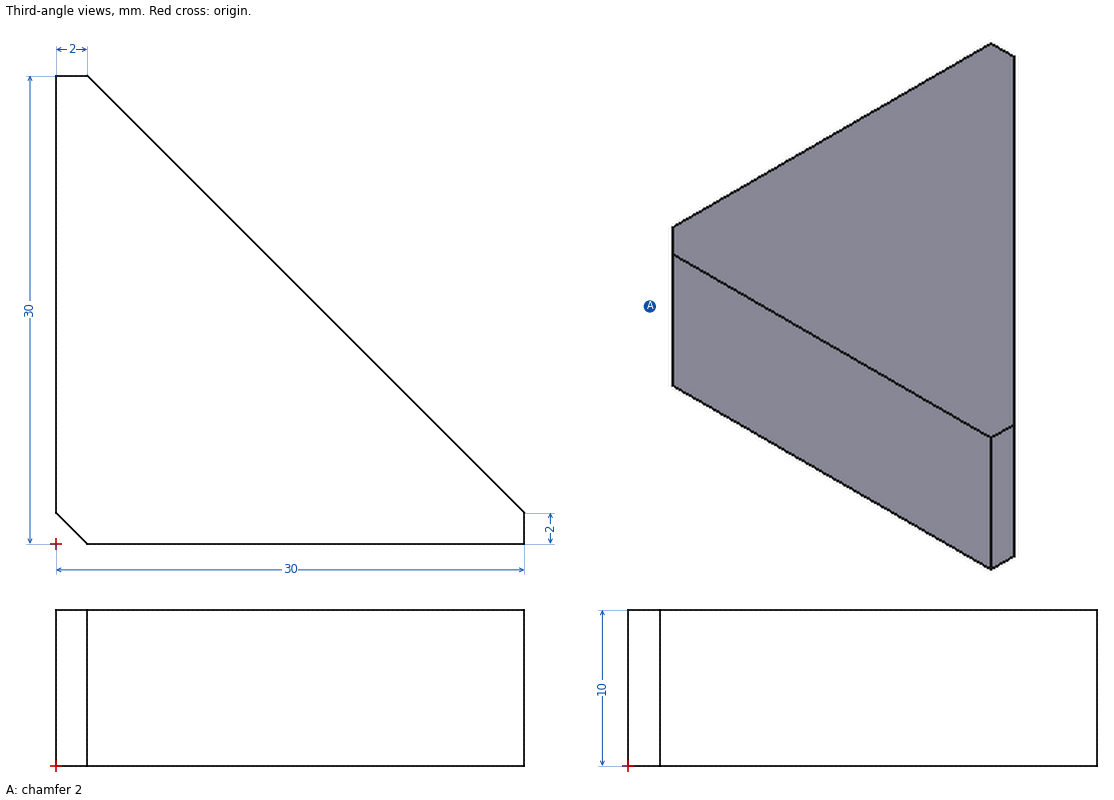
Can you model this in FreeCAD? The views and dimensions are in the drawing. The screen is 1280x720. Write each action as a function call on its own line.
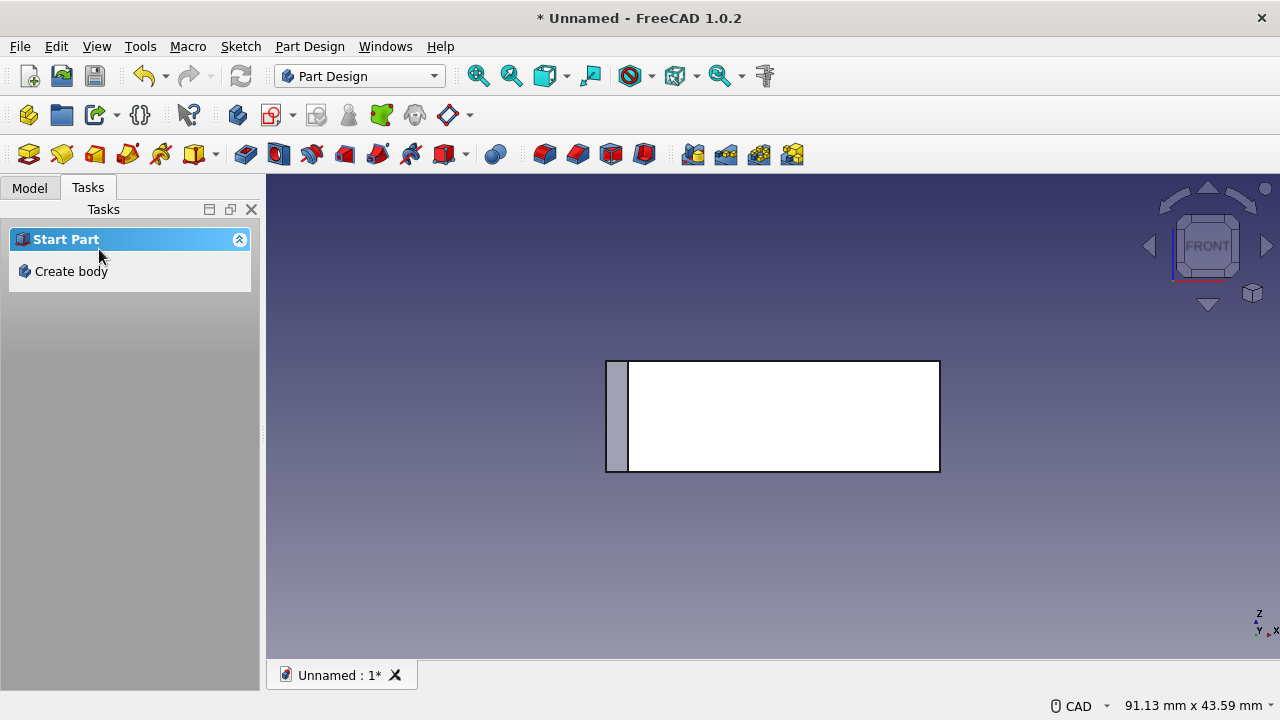
key(0)